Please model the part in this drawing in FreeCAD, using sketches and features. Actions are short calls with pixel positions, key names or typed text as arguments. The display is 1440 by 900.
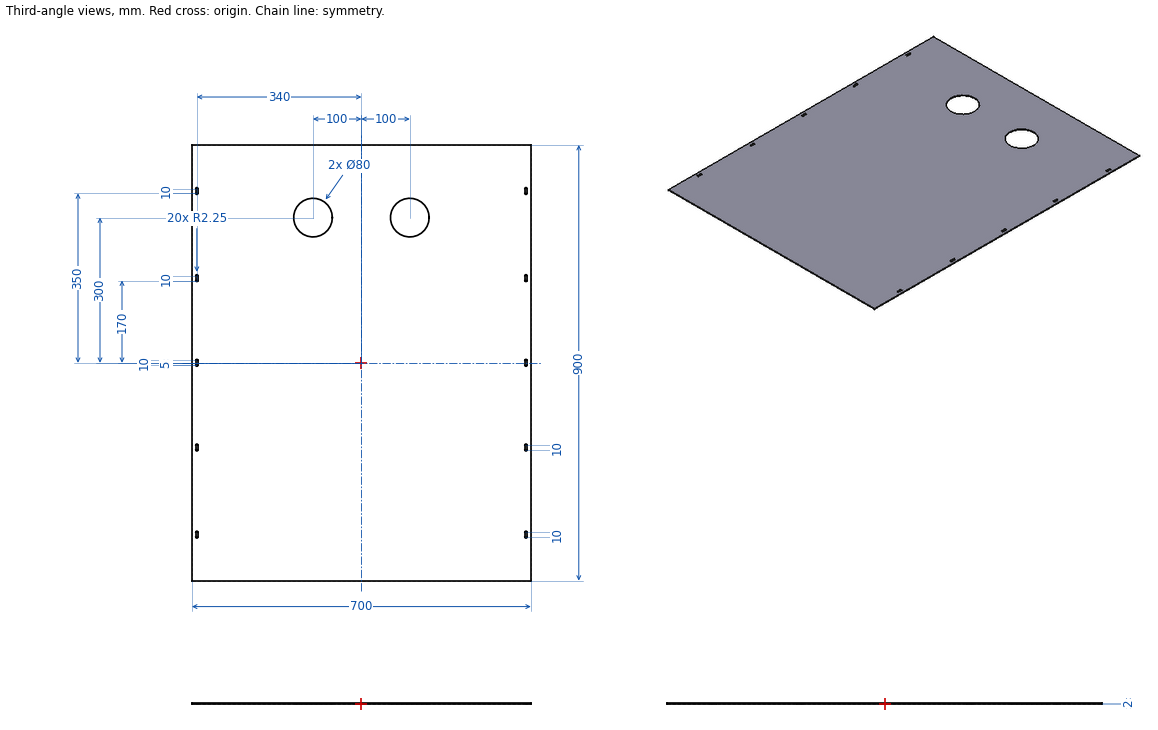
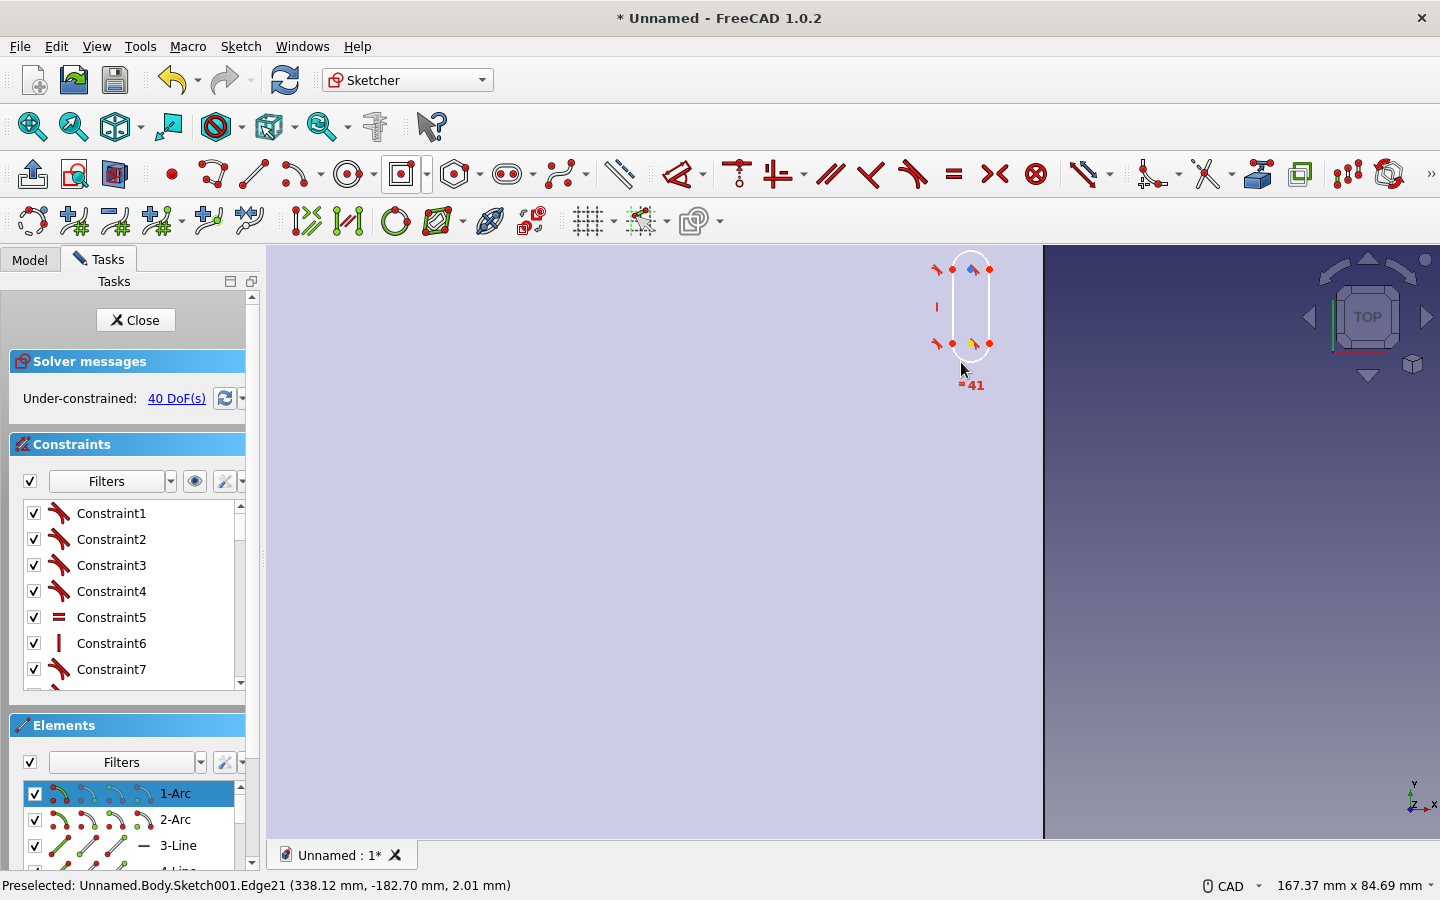
click(960, 358)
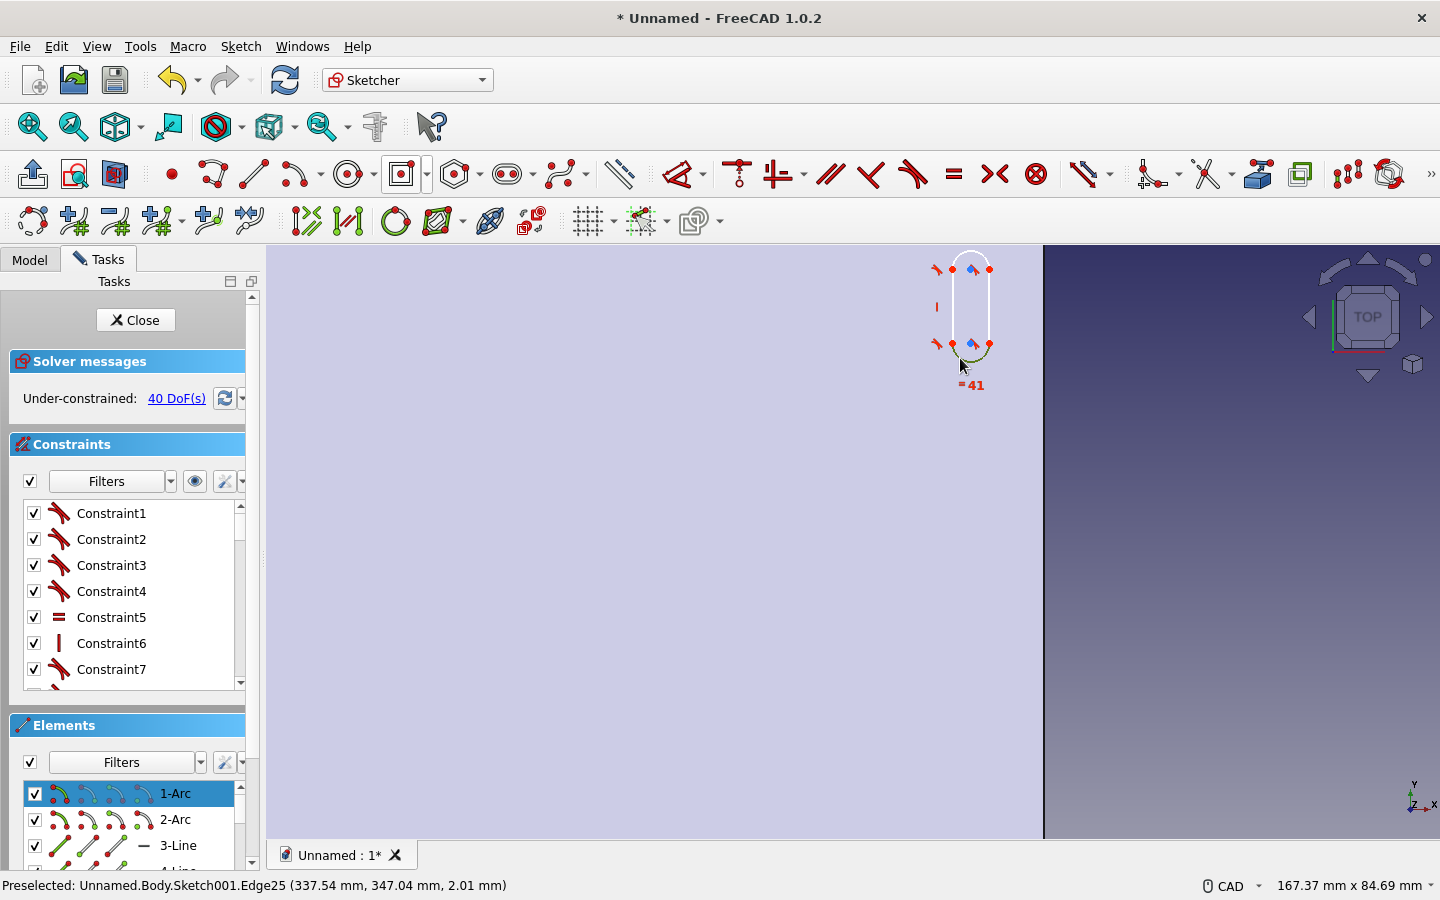
scroll(961, 362, down, 13)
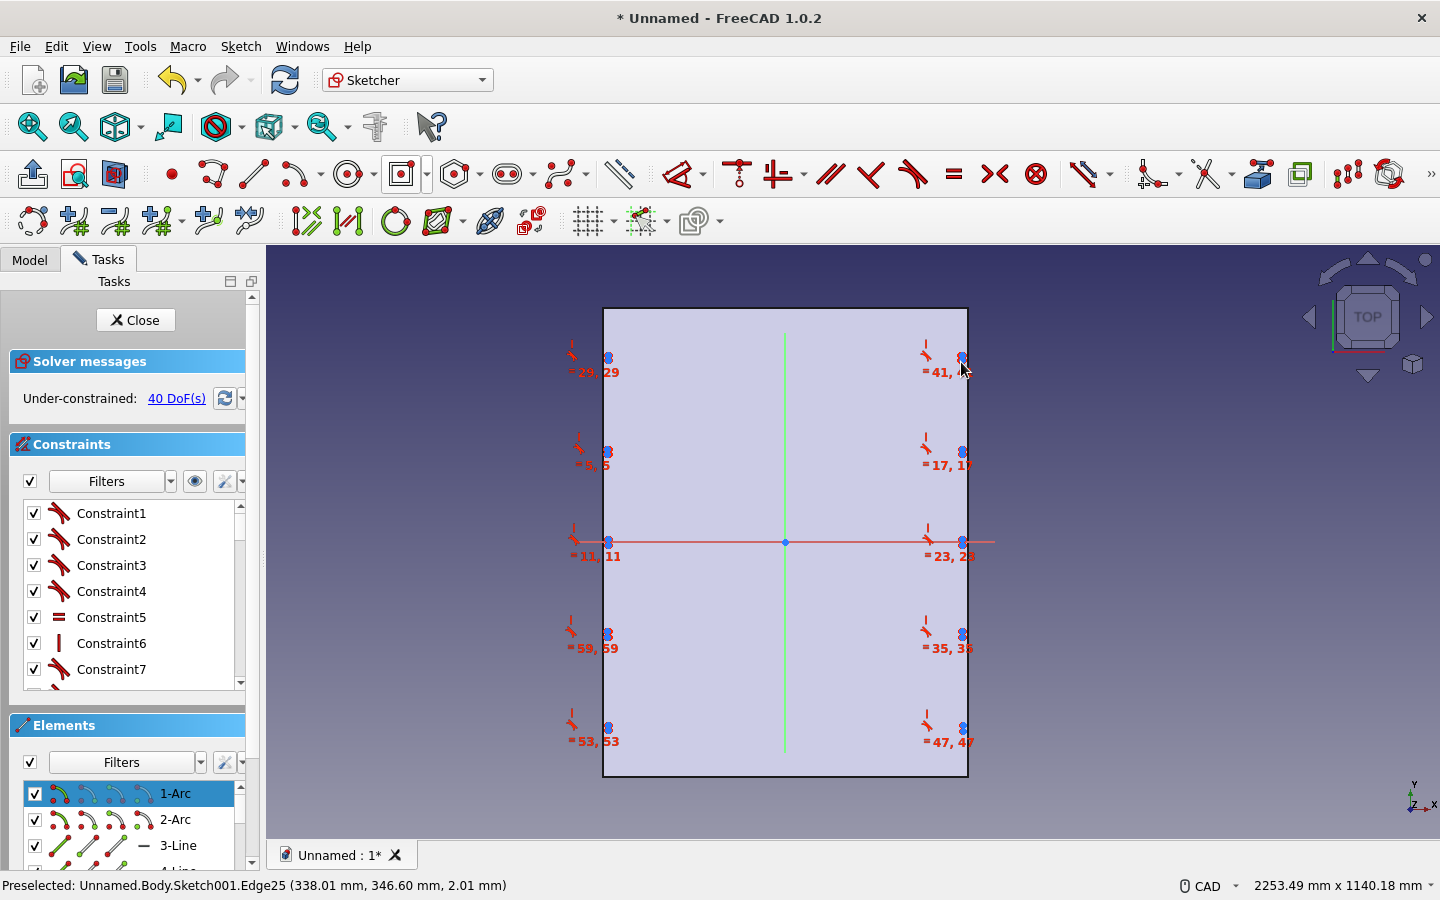
scroll(963, 732, up, 14)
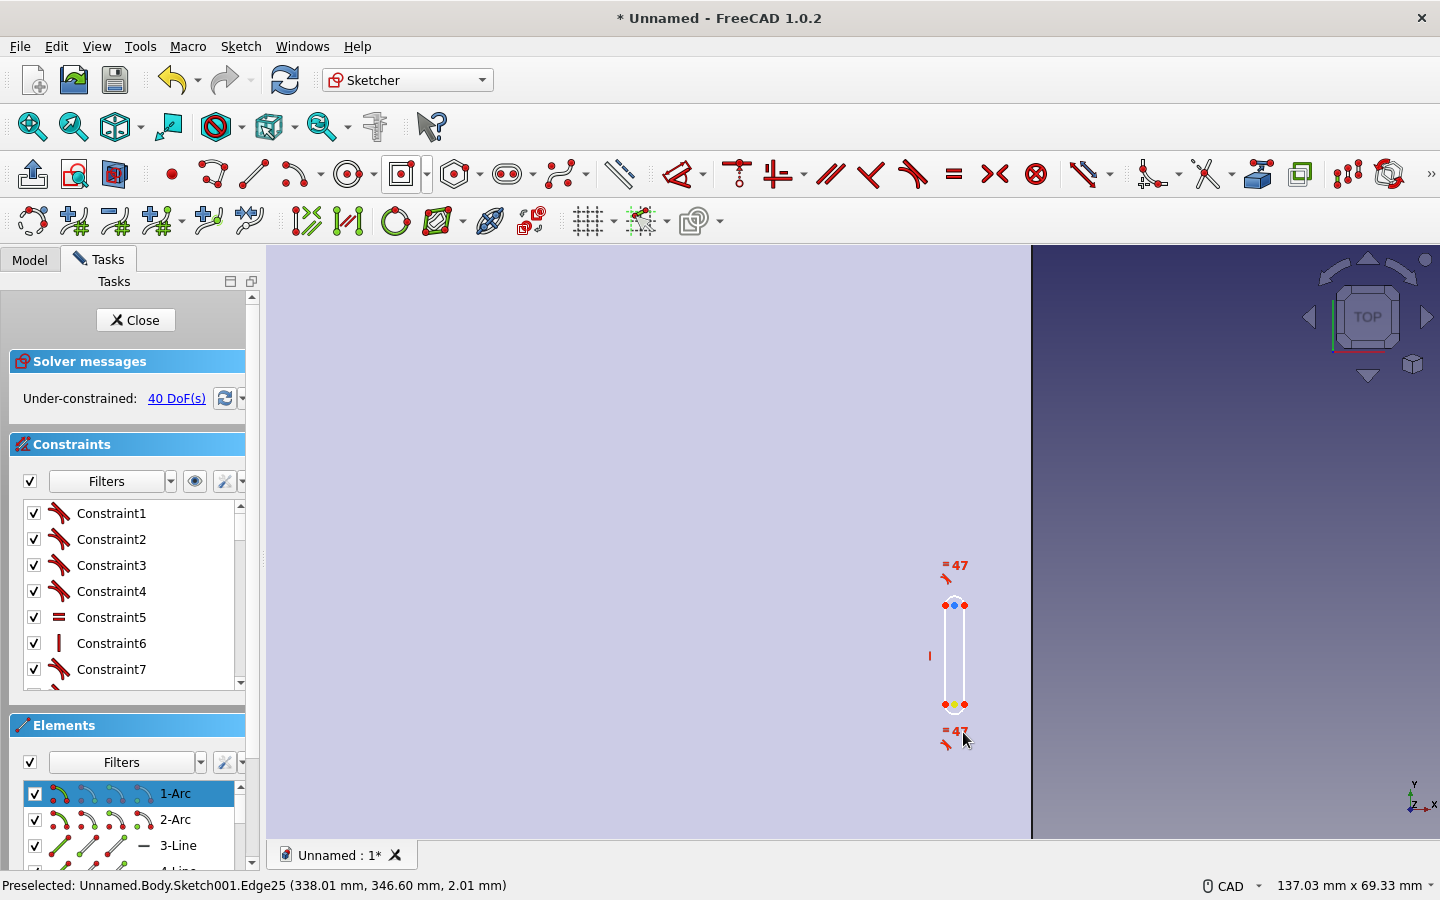
click(955, 714)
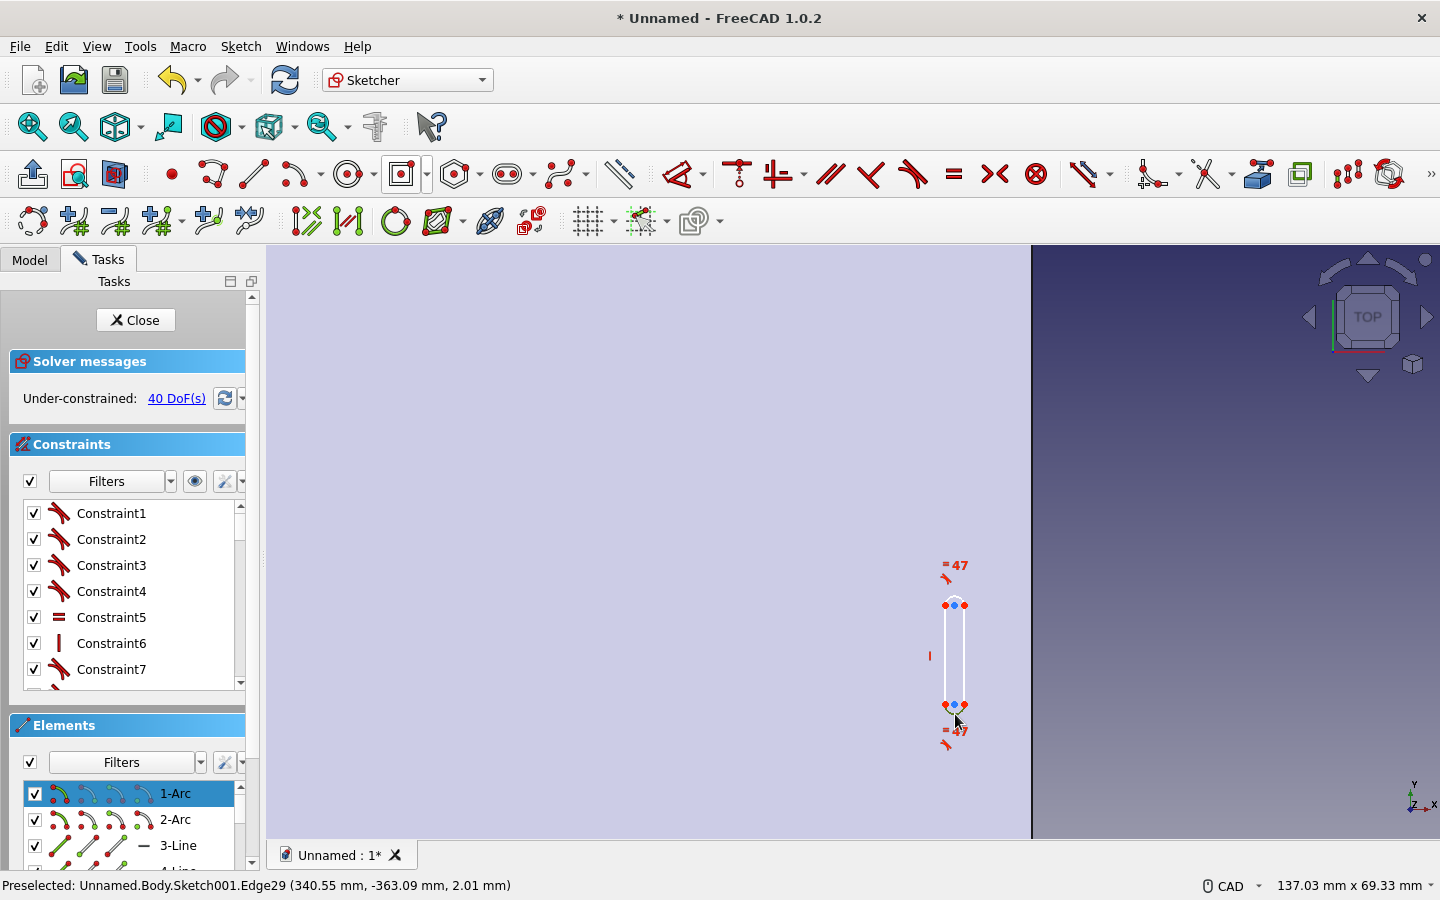
scroll(963, 732, down, 14)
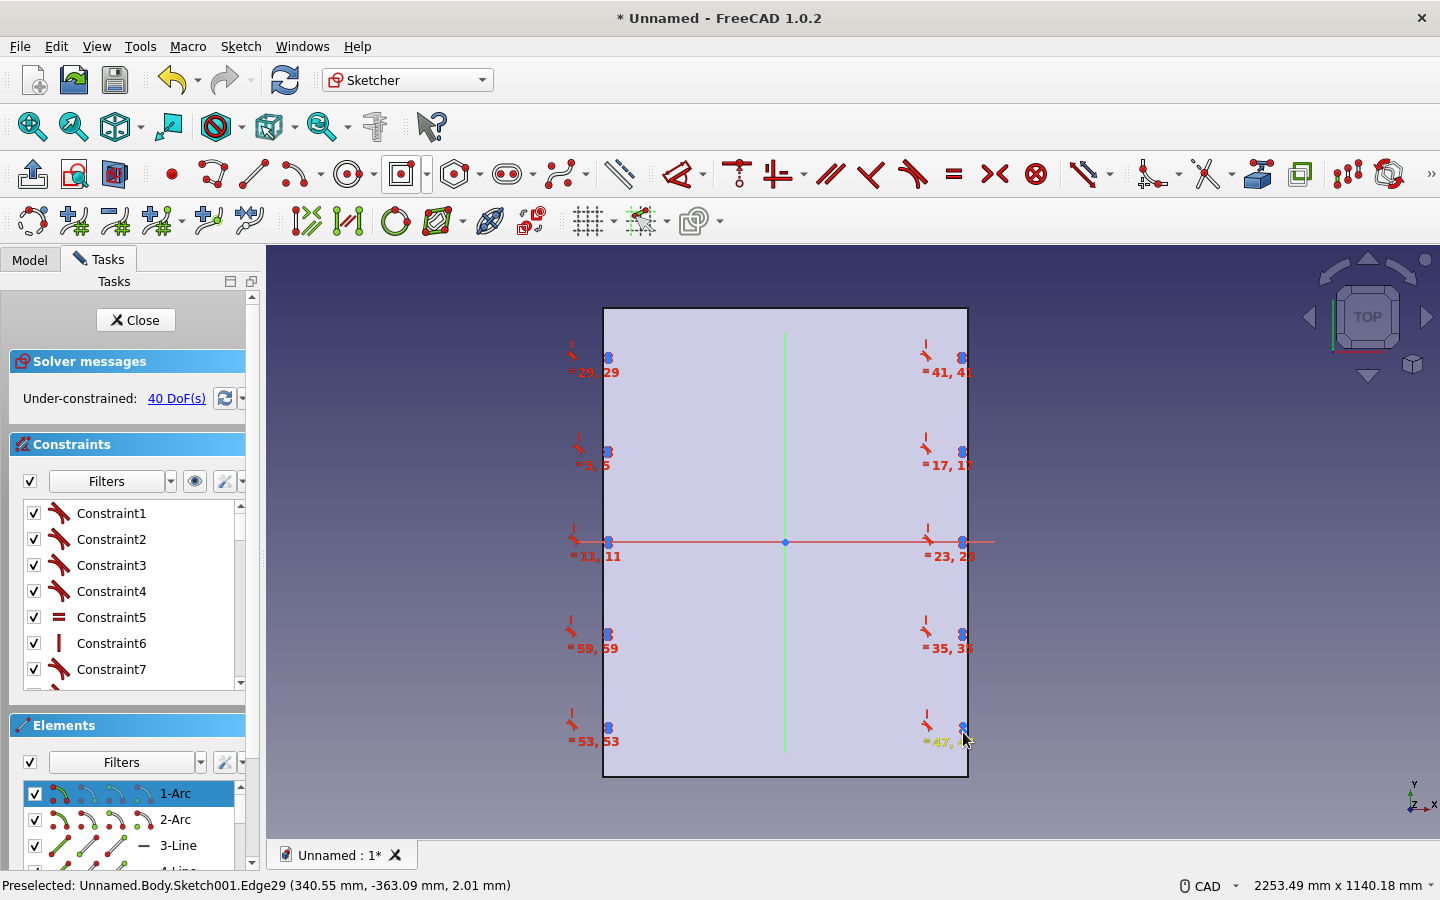
scroll(608, 732, up, 14)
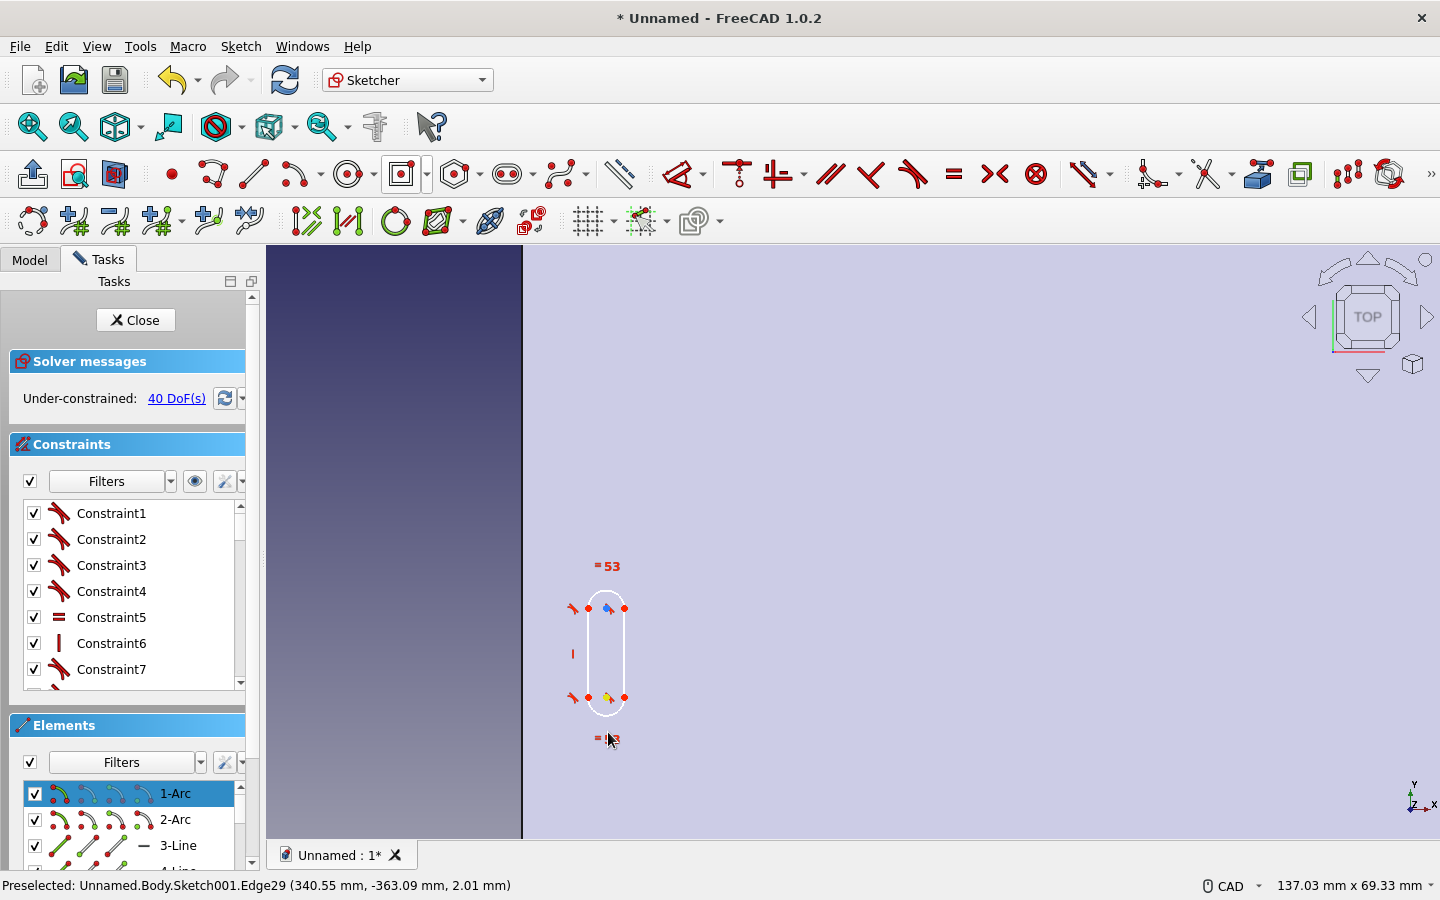
click(596, 712)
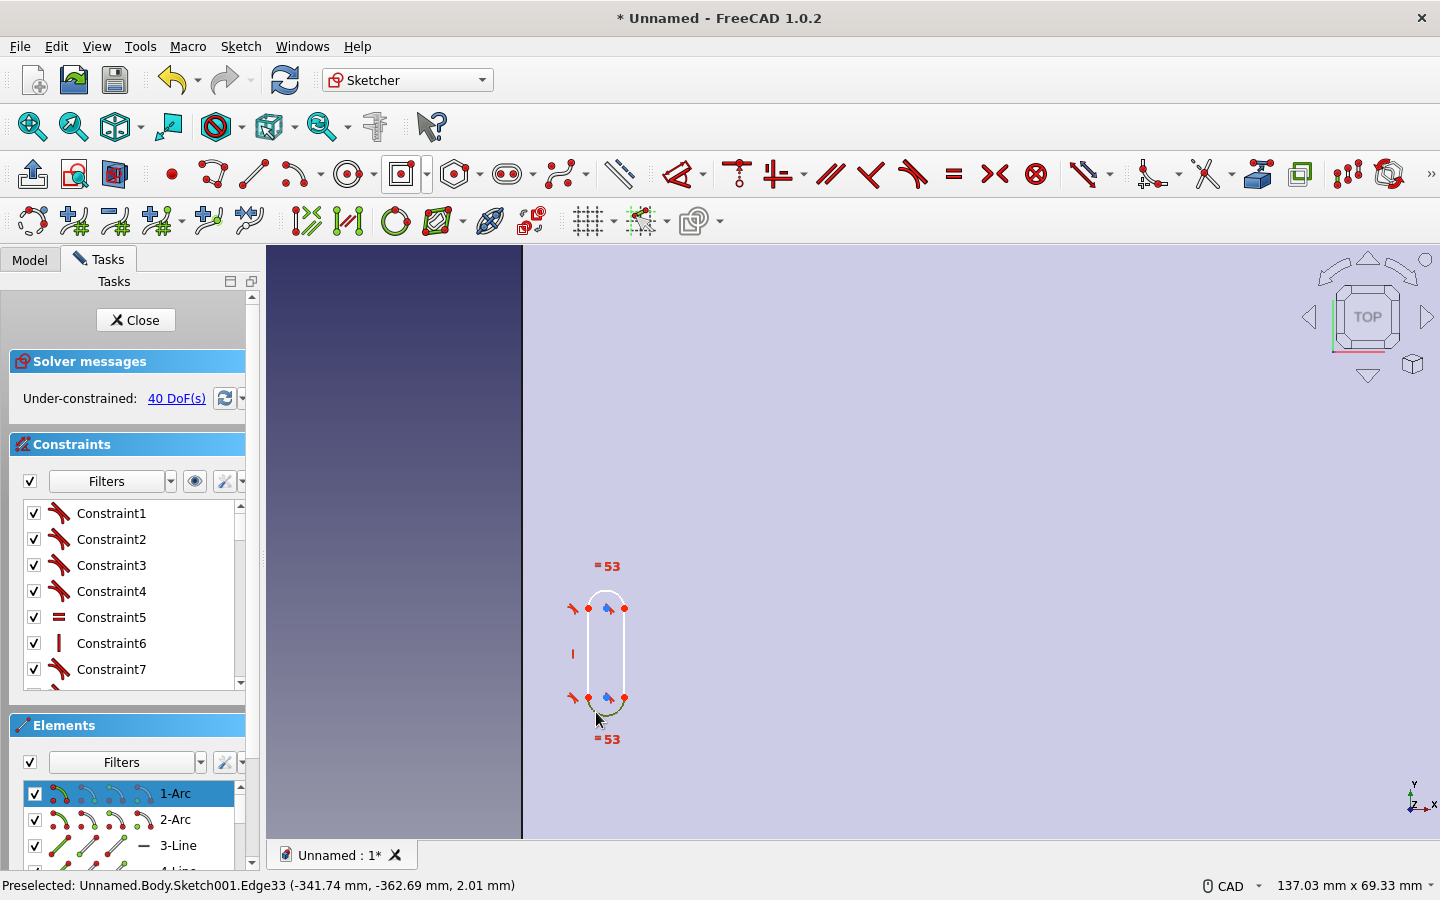
scroll(607, 732, down, 14)